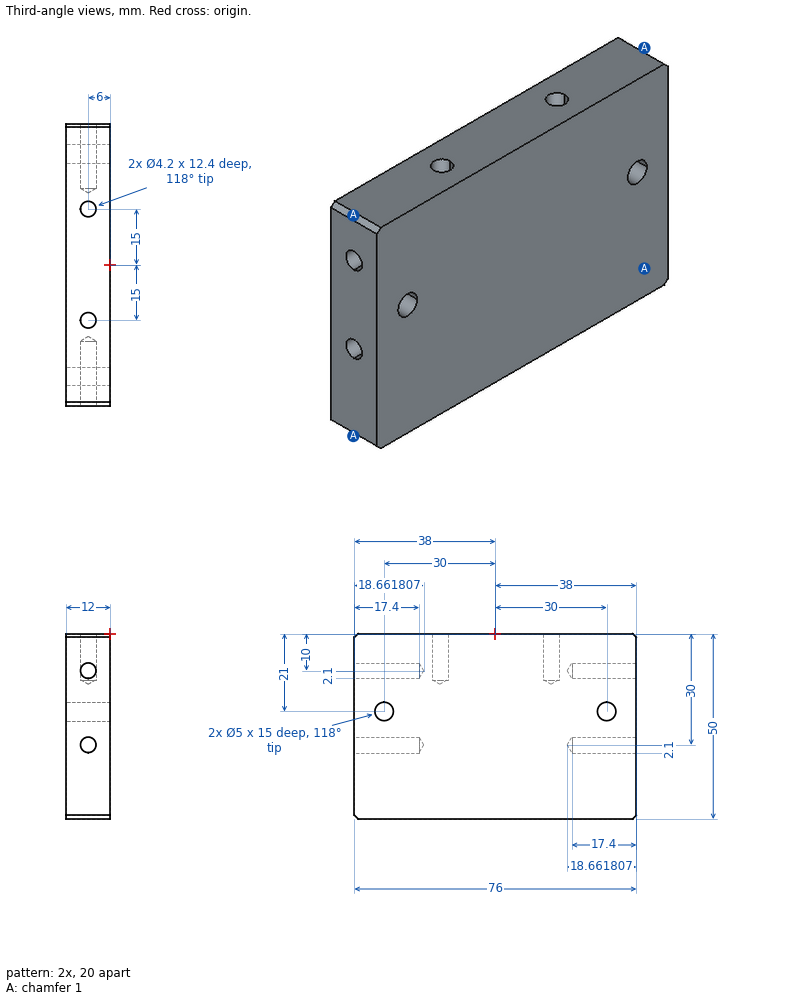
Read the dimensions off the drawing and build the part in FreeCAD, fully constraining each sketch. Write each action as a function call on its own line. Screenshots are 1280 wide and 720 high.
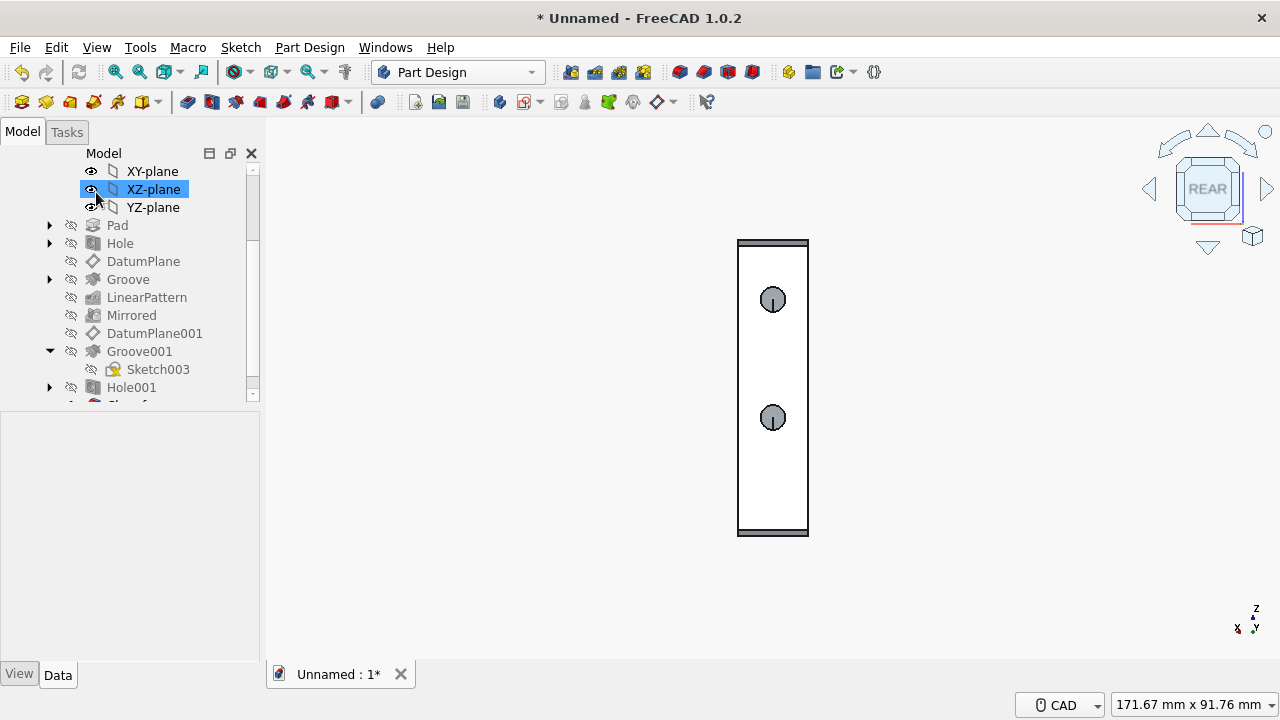
key(0)